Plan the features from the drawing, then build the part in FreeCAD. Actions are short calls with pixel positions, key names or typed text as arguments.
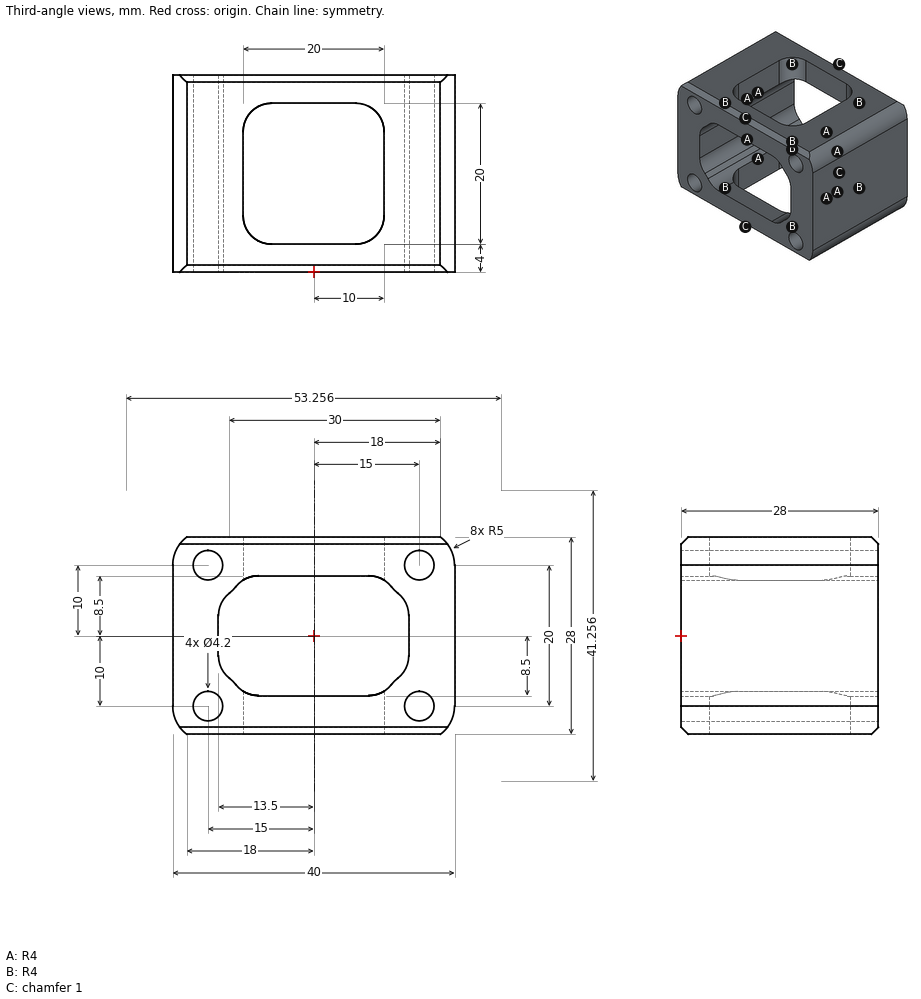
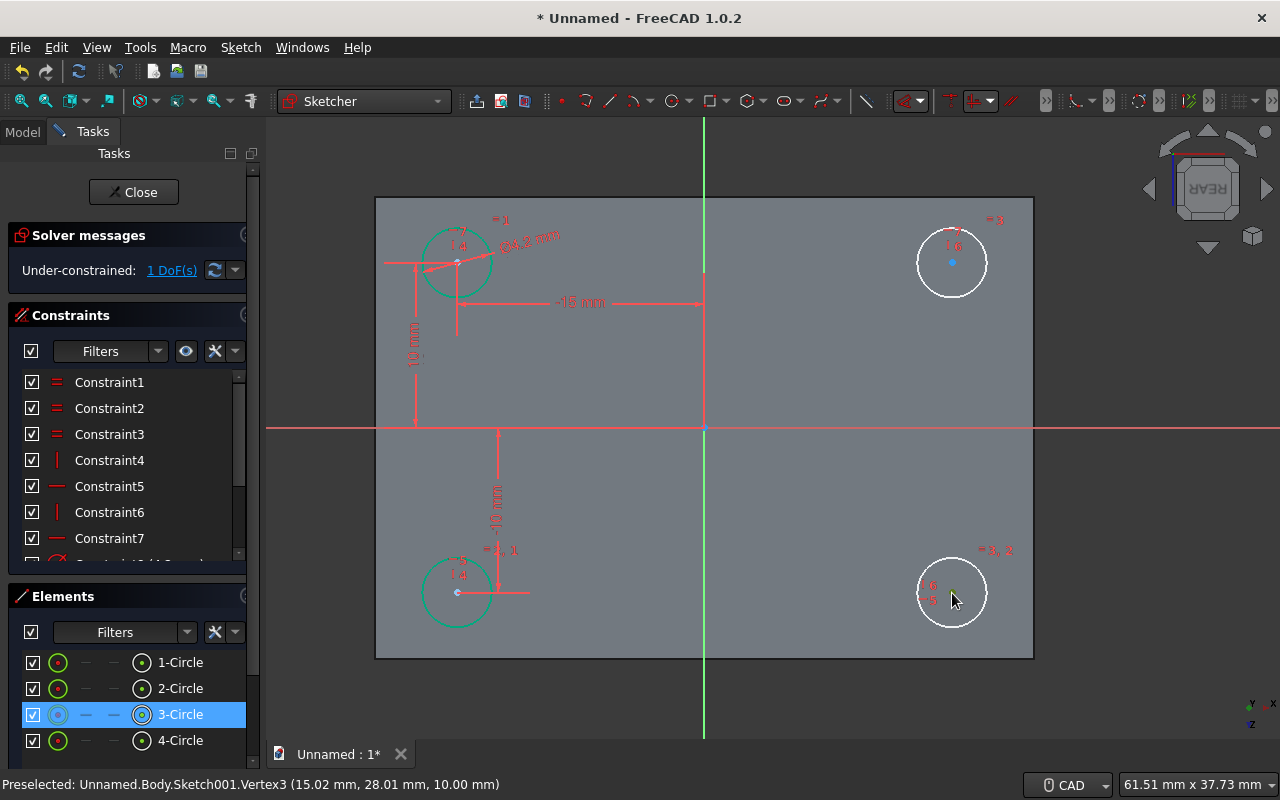
key(l)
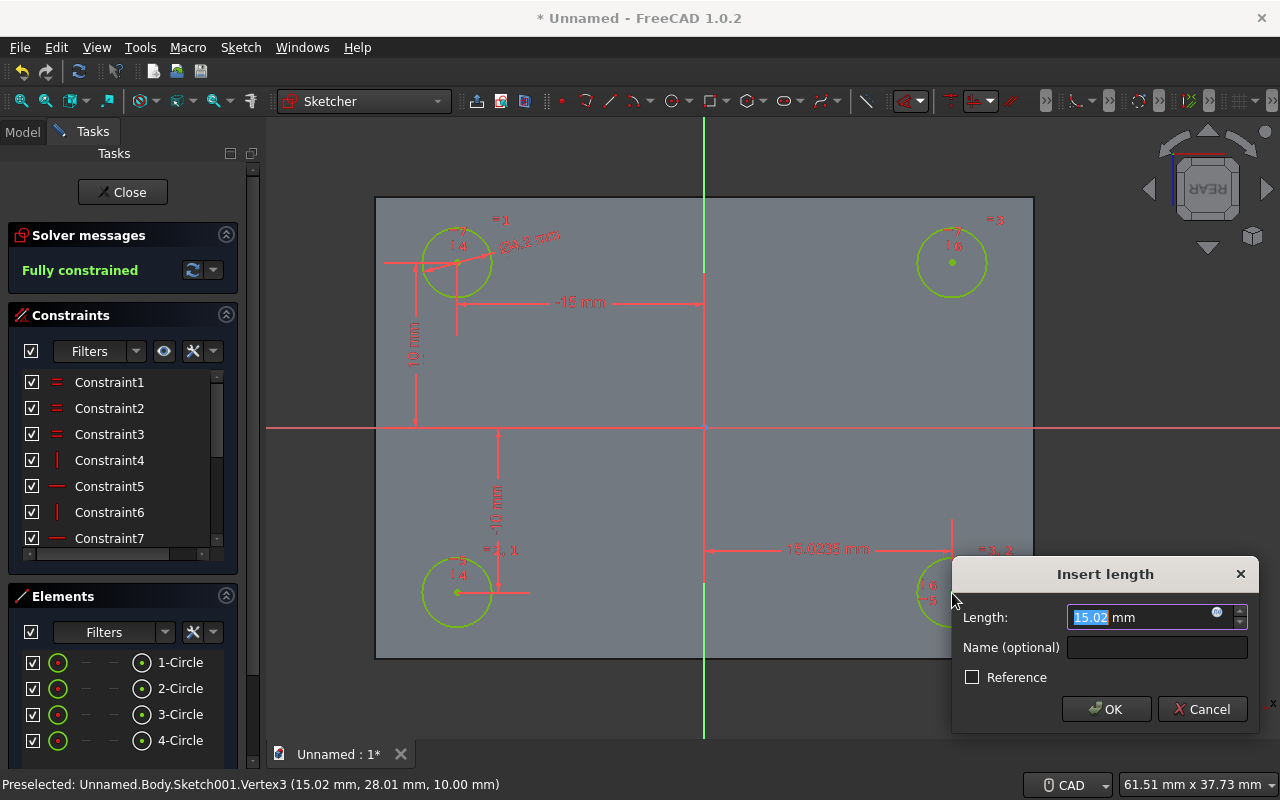
text(15)
key(Return)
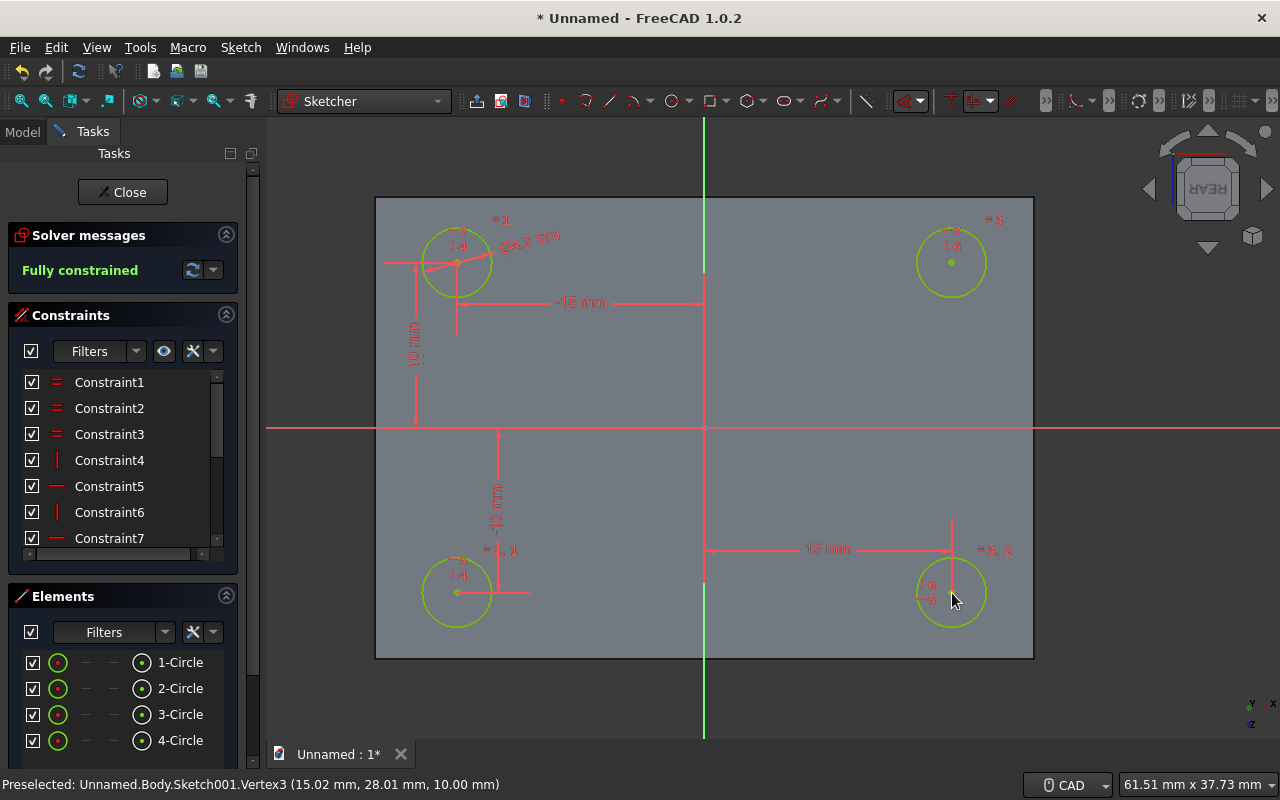
click(123, 192)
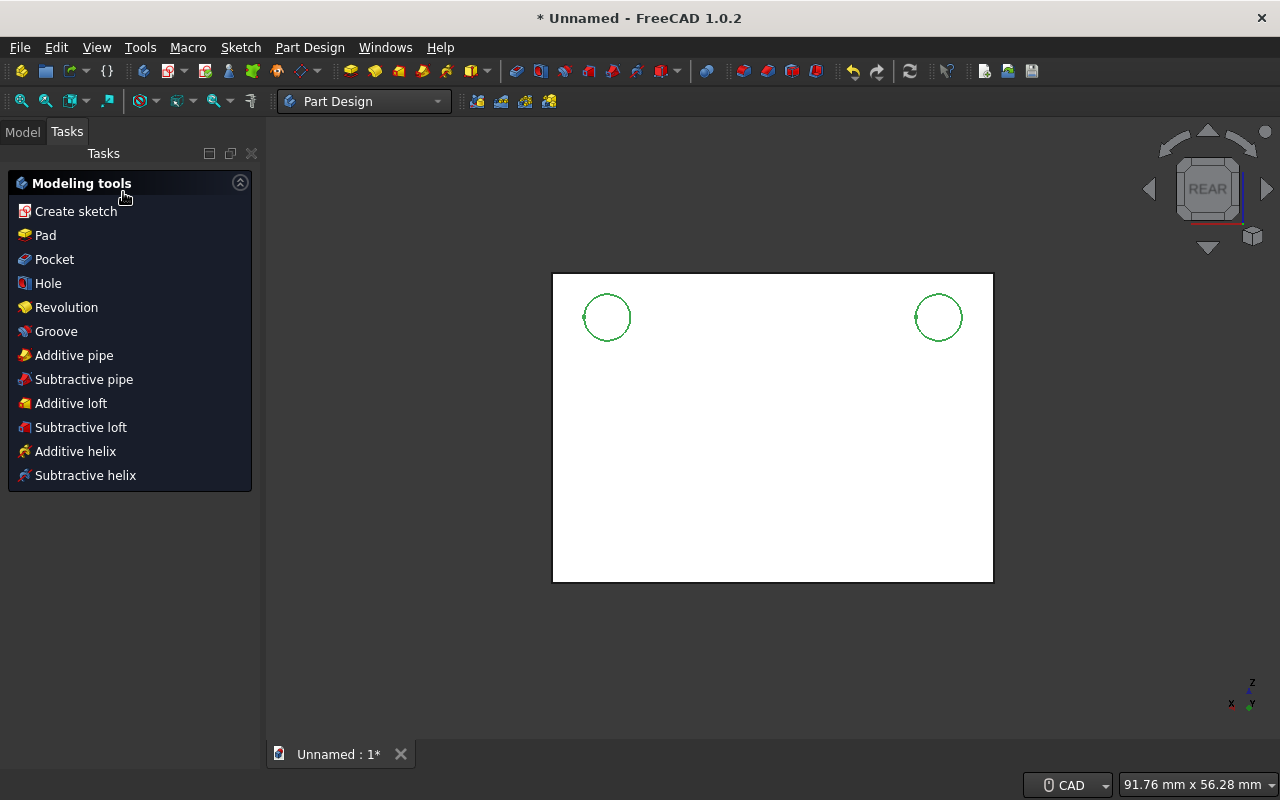
click(518, 72)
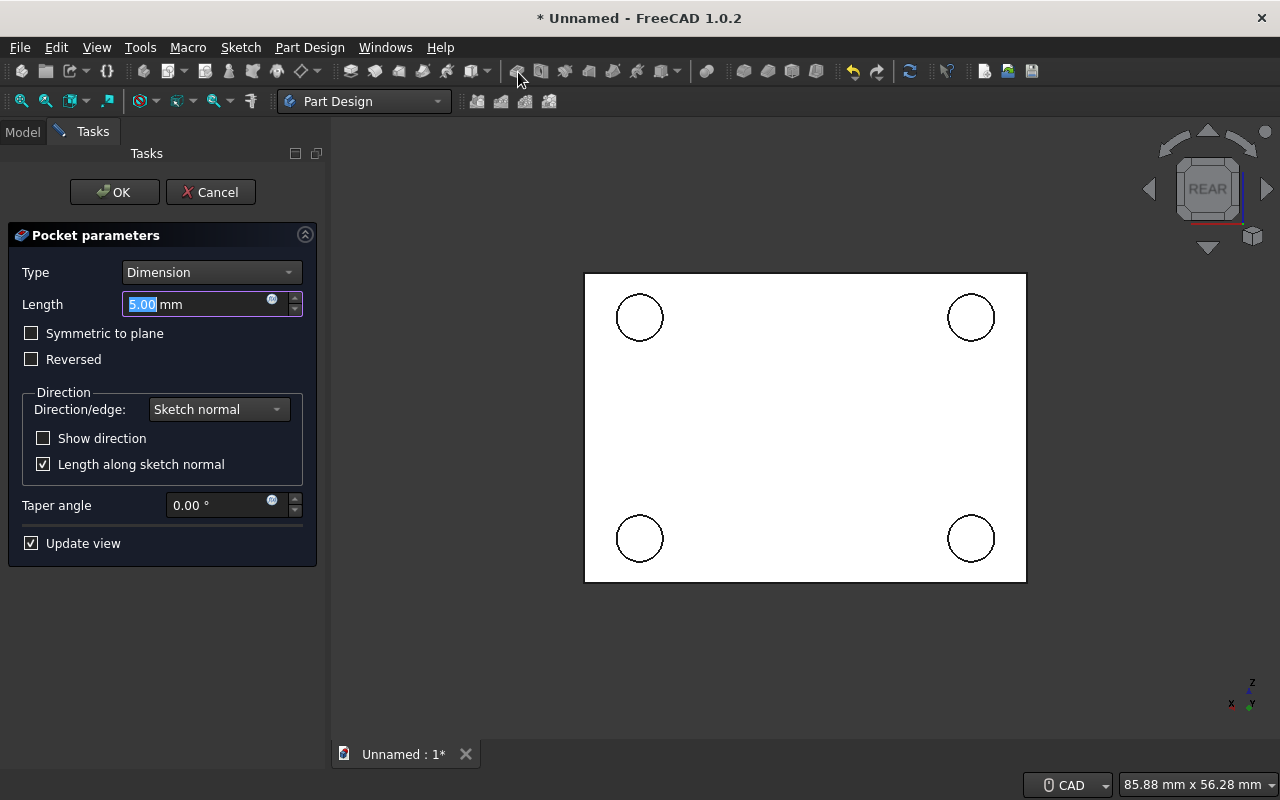
click(212, 272)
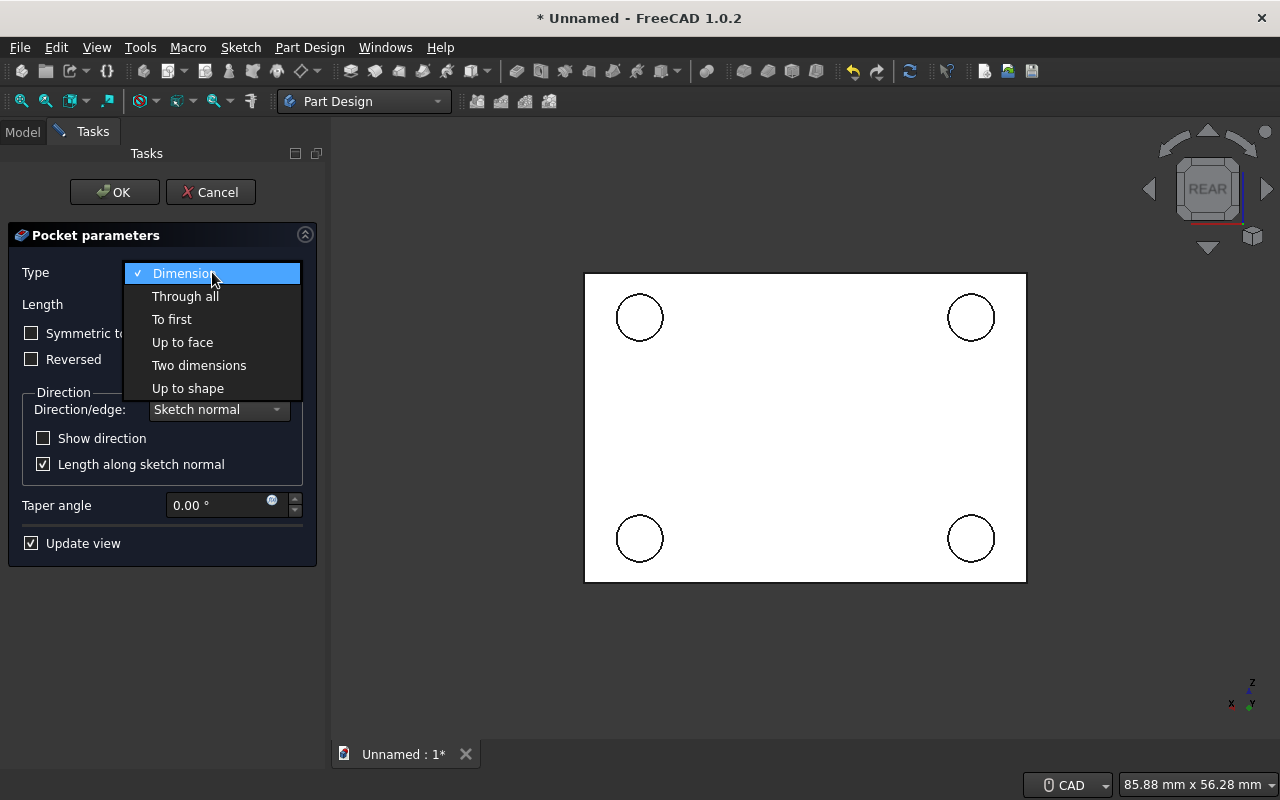
click(212, 296)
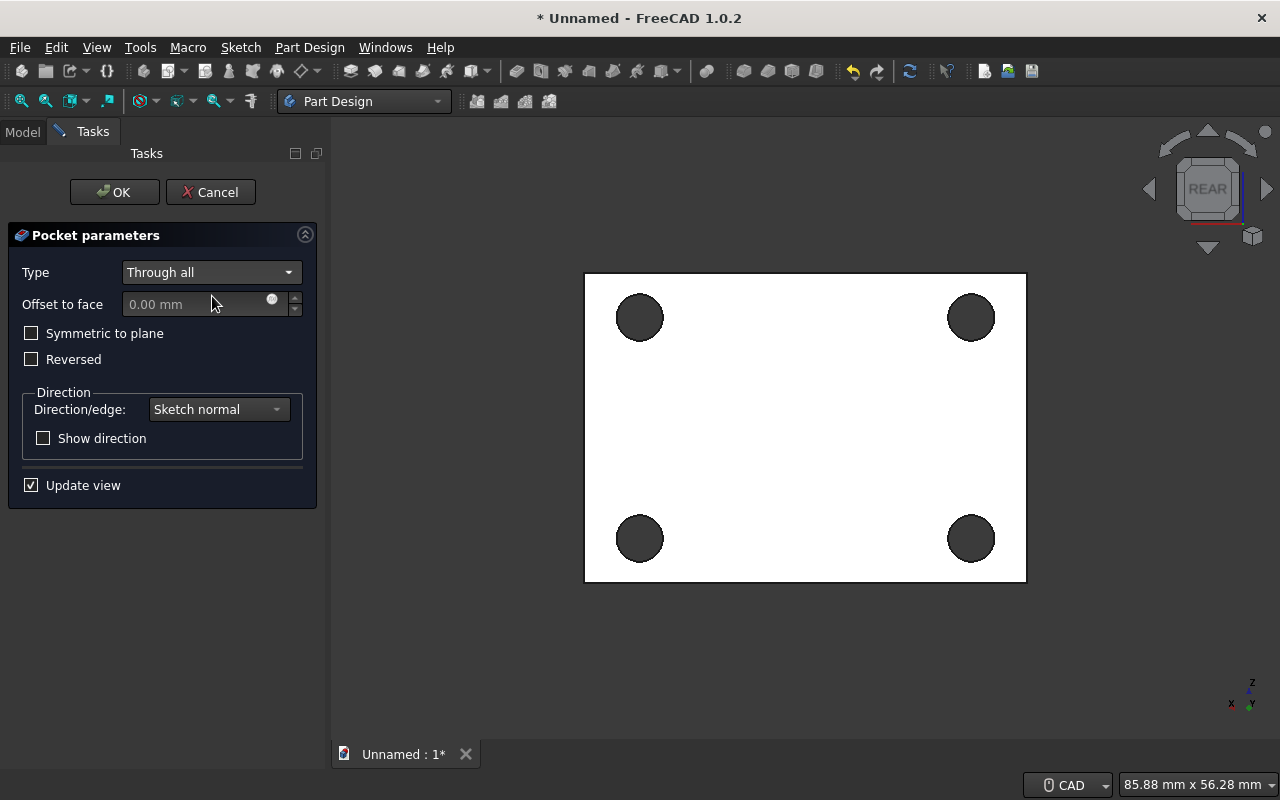
click(115, 192)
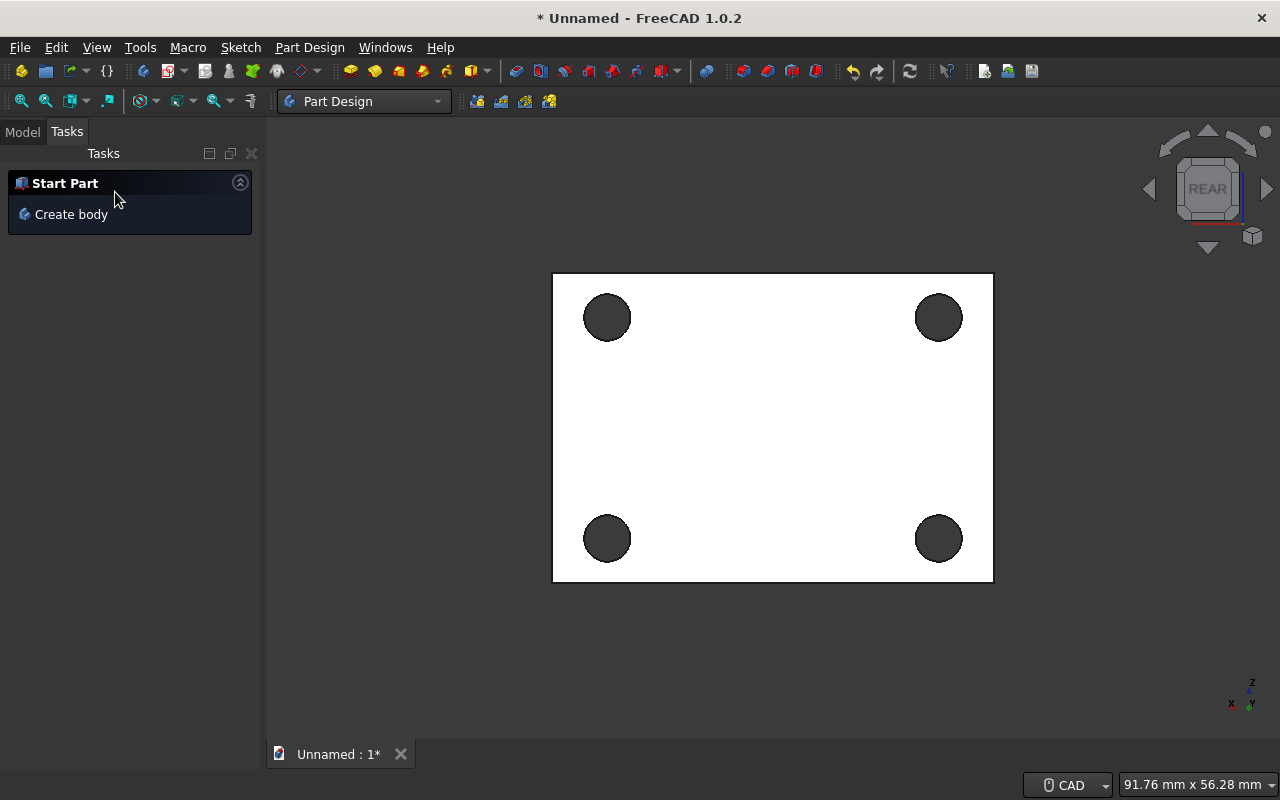
click(773, 427)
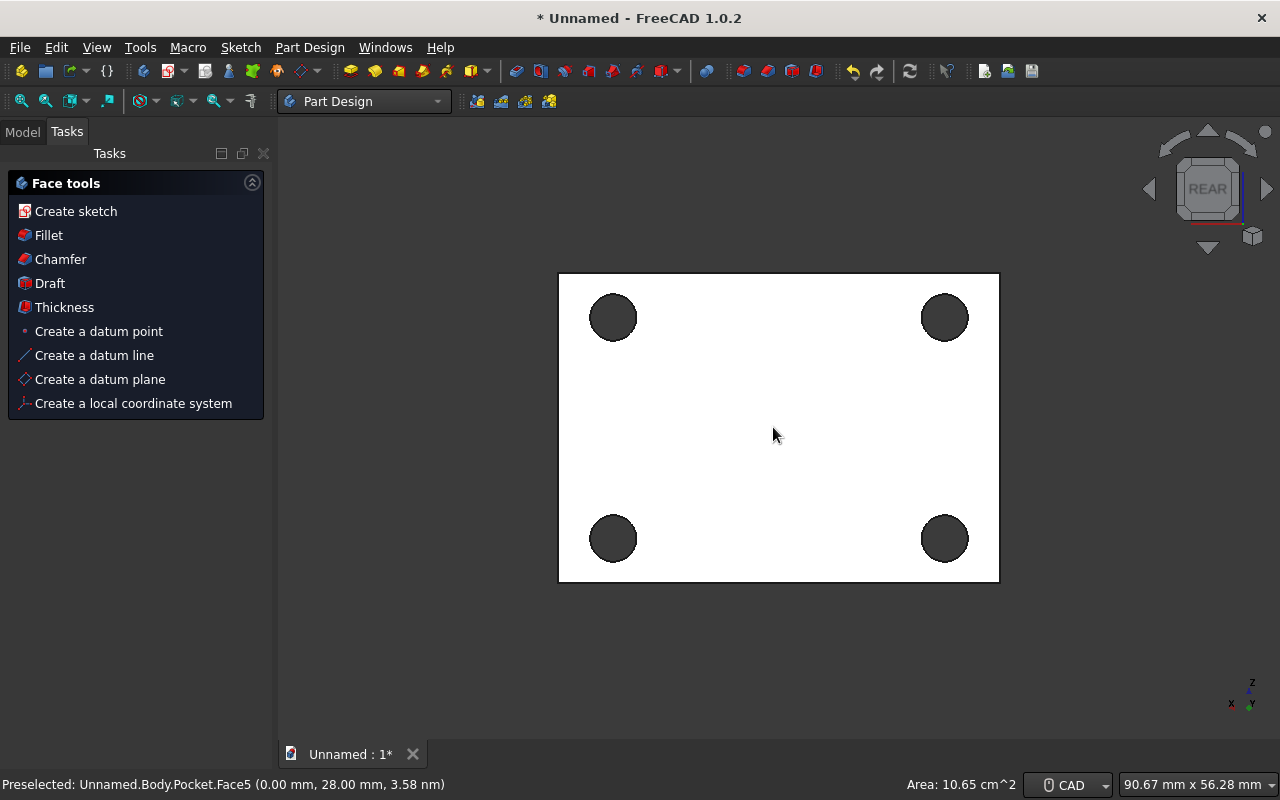
click(168, 72)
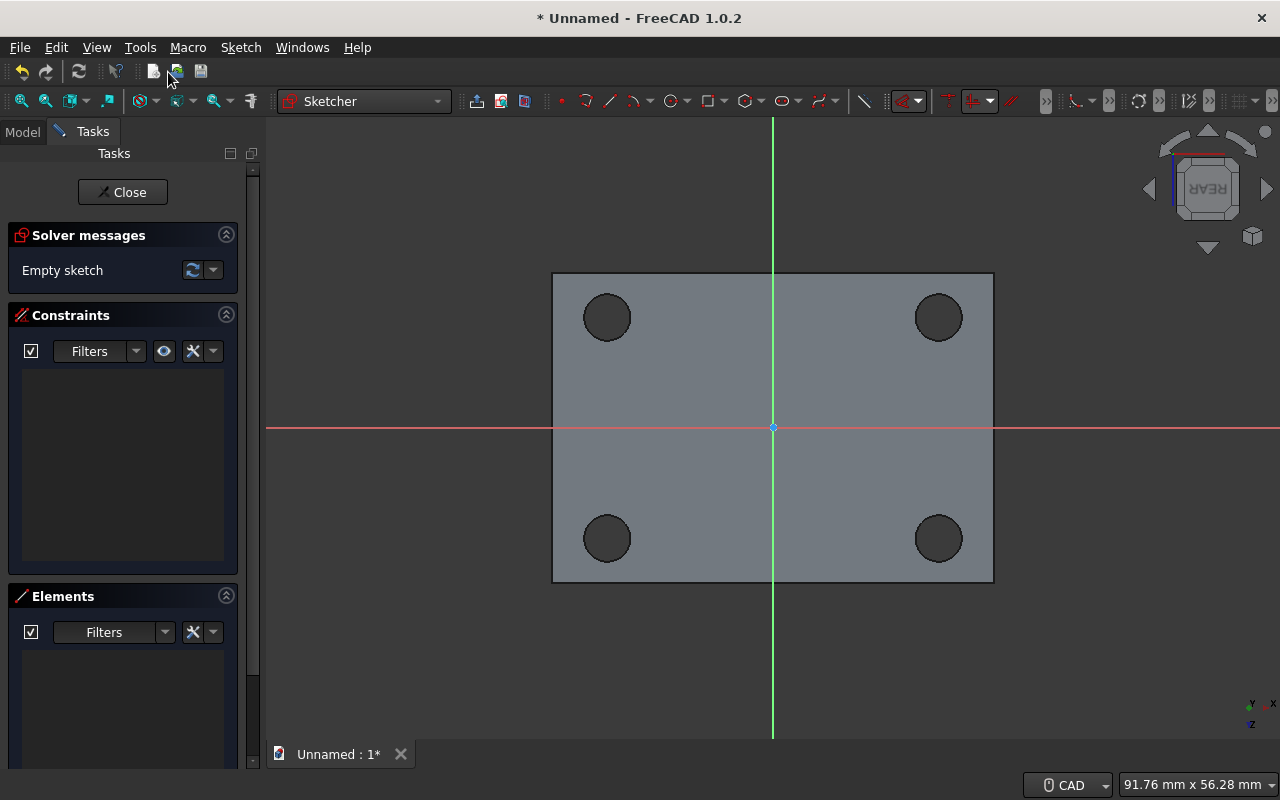
key(g)
key(v)